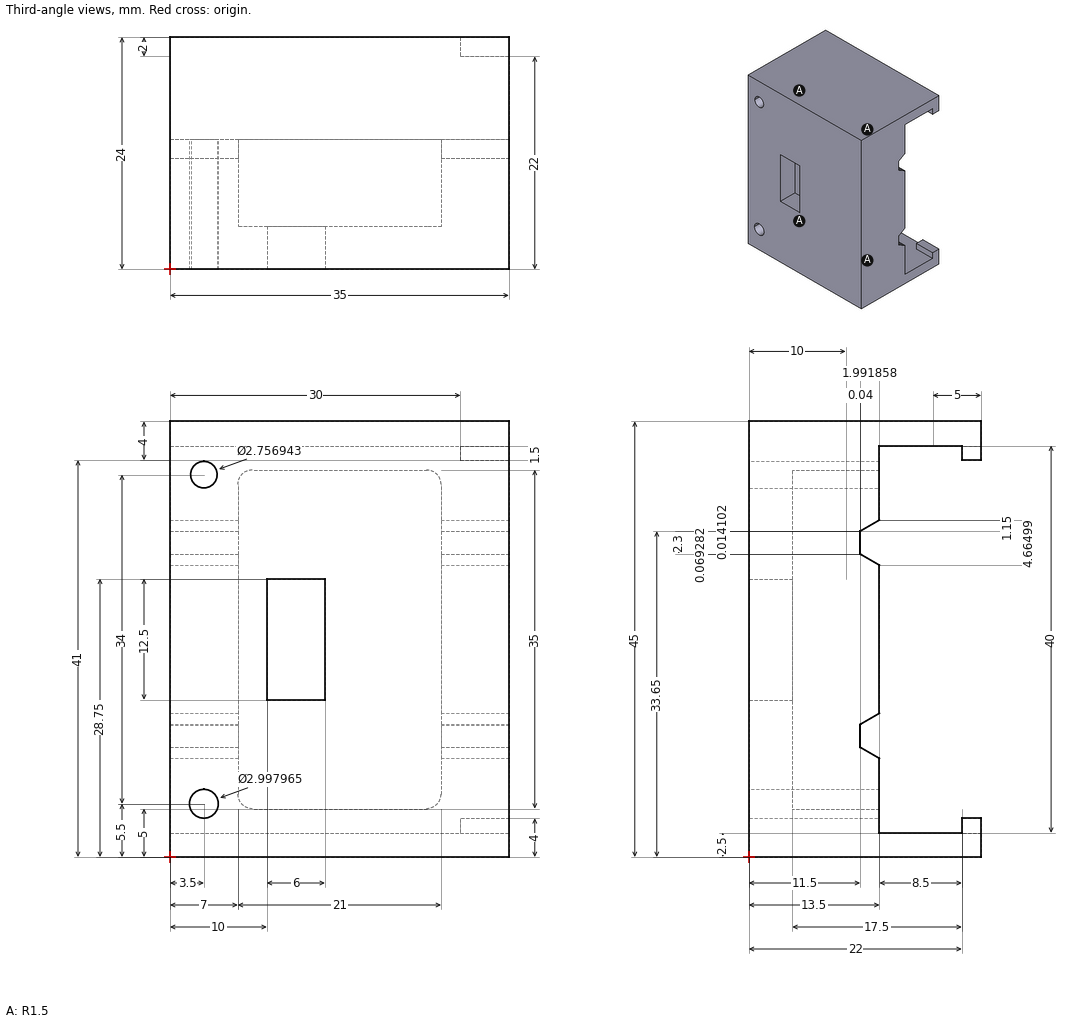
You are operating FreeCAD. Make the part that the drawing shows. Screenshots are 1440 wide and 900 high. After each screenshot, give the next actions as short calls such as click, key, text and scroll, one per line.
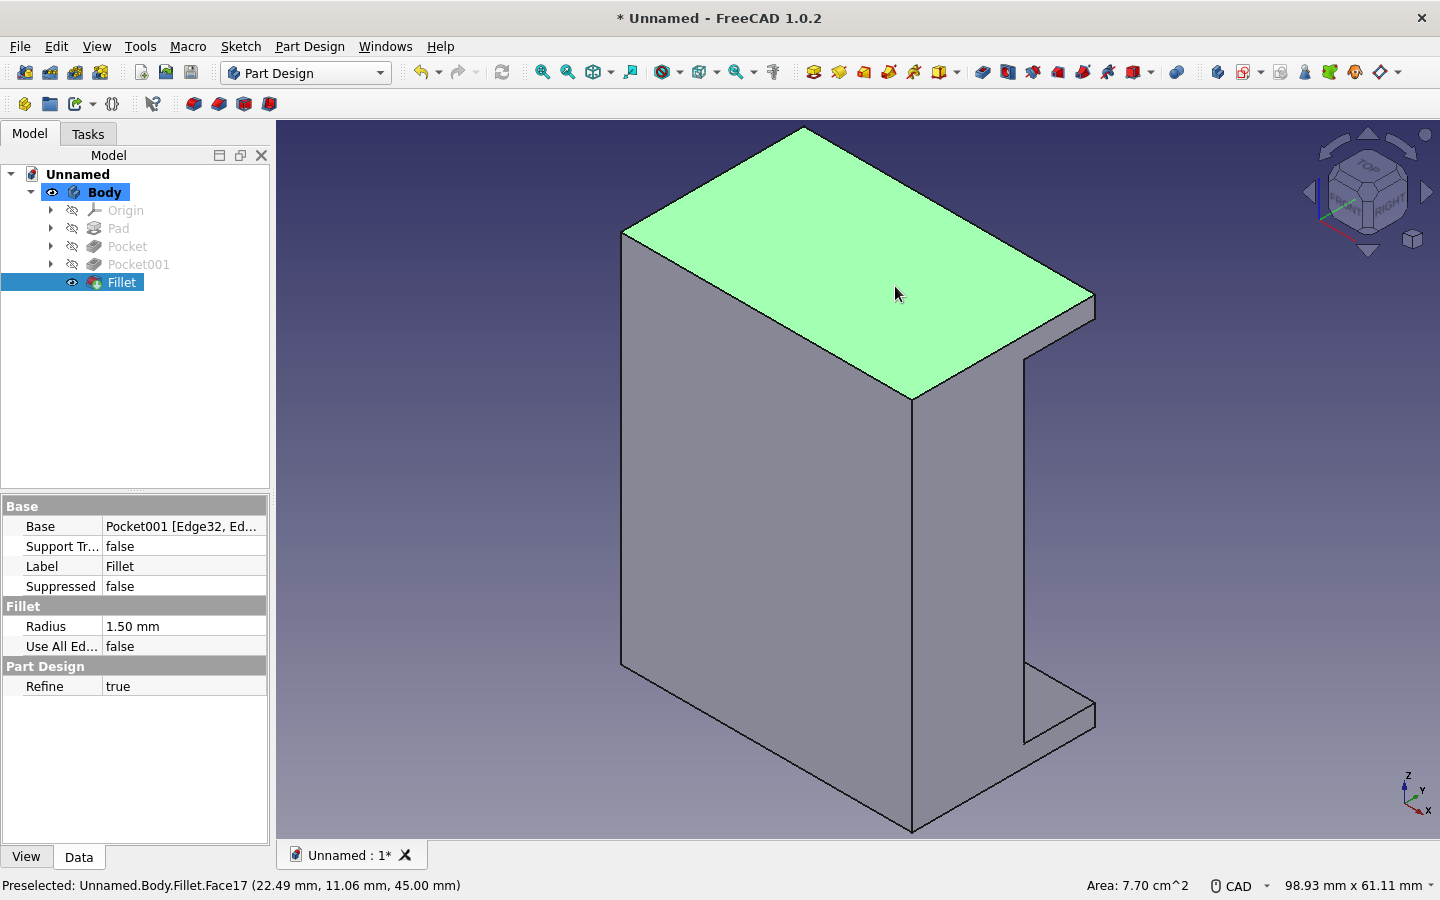
click(1242, 72)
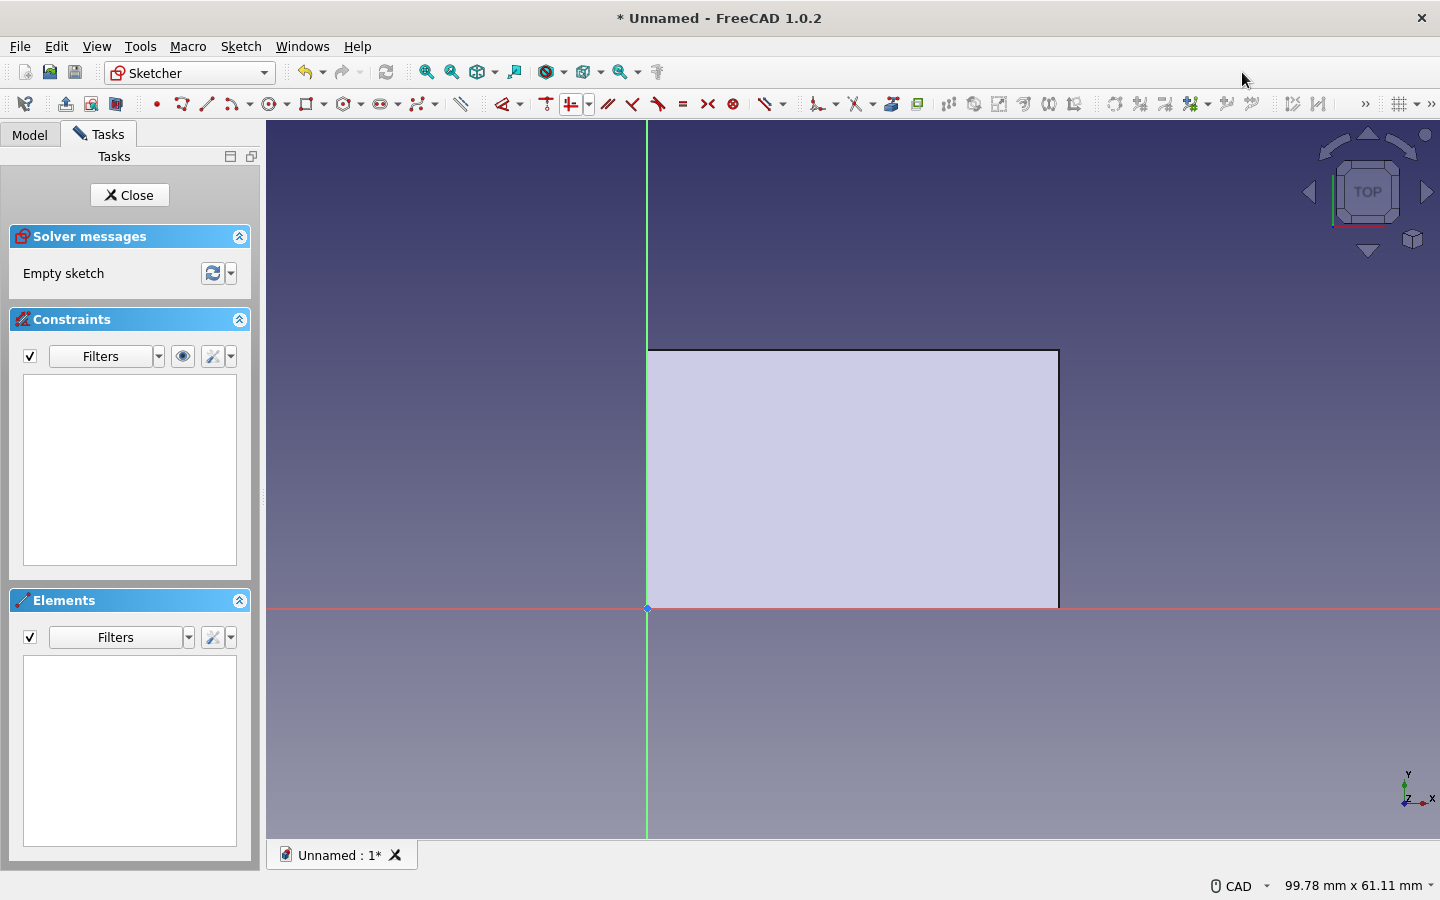
scroll(936, 453, up, 3)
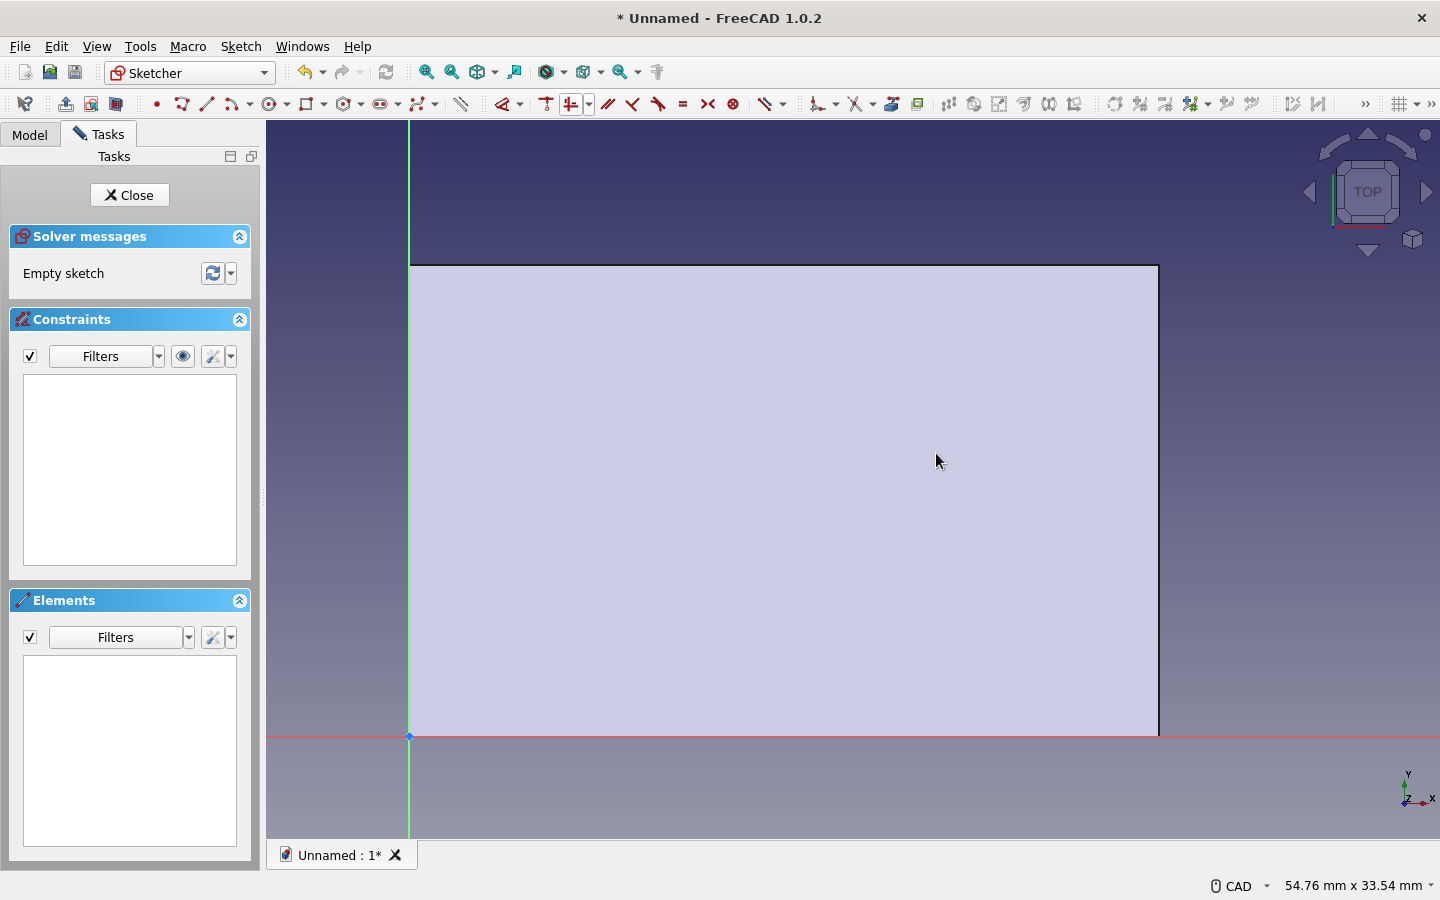
click(306, 104)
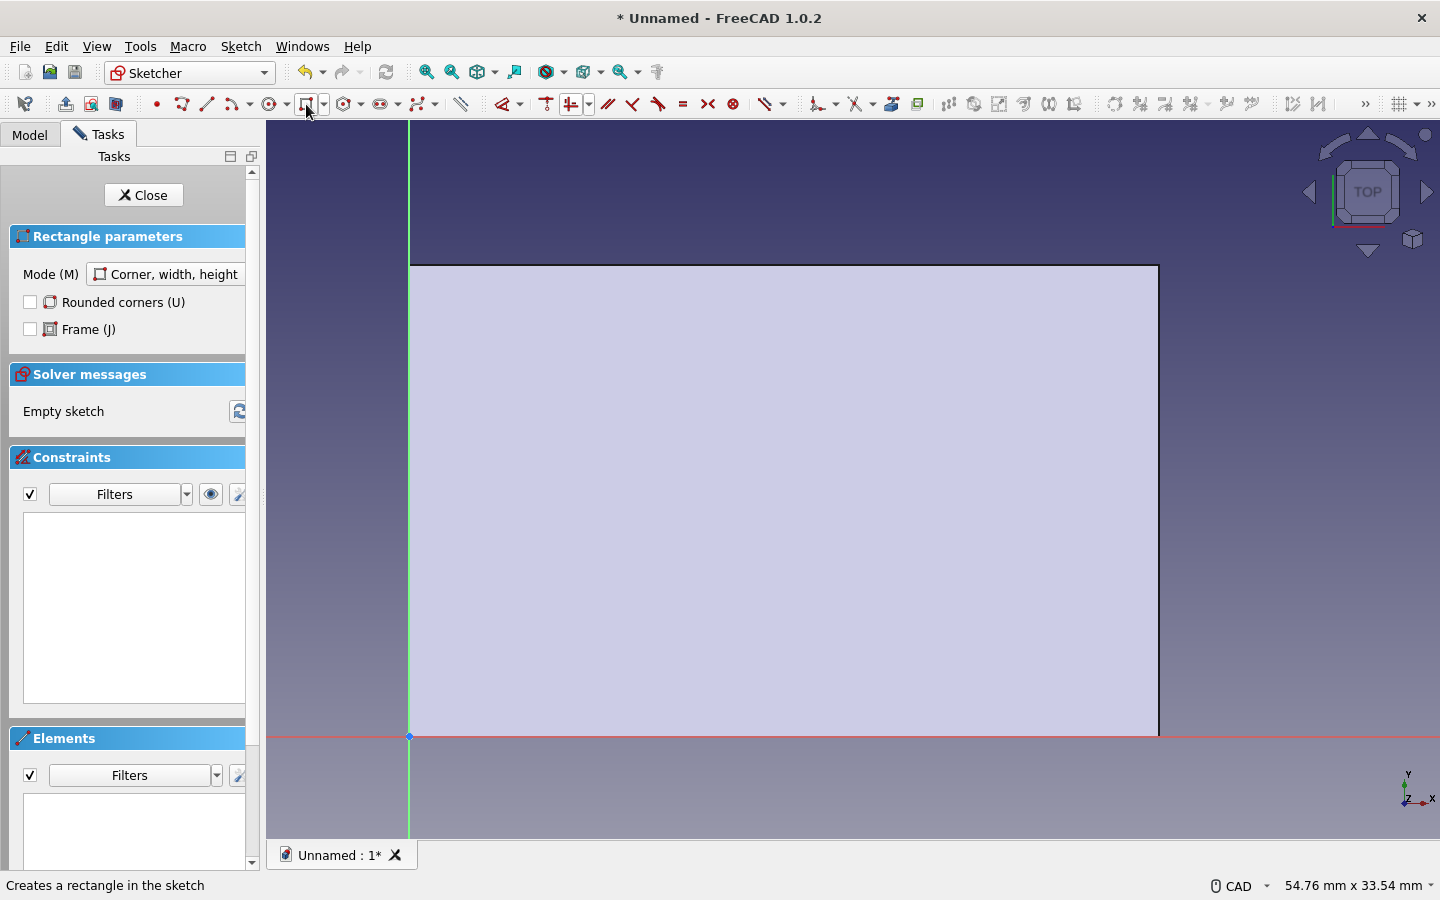
click(409, 222)
click(1159, 265)
key(Escape)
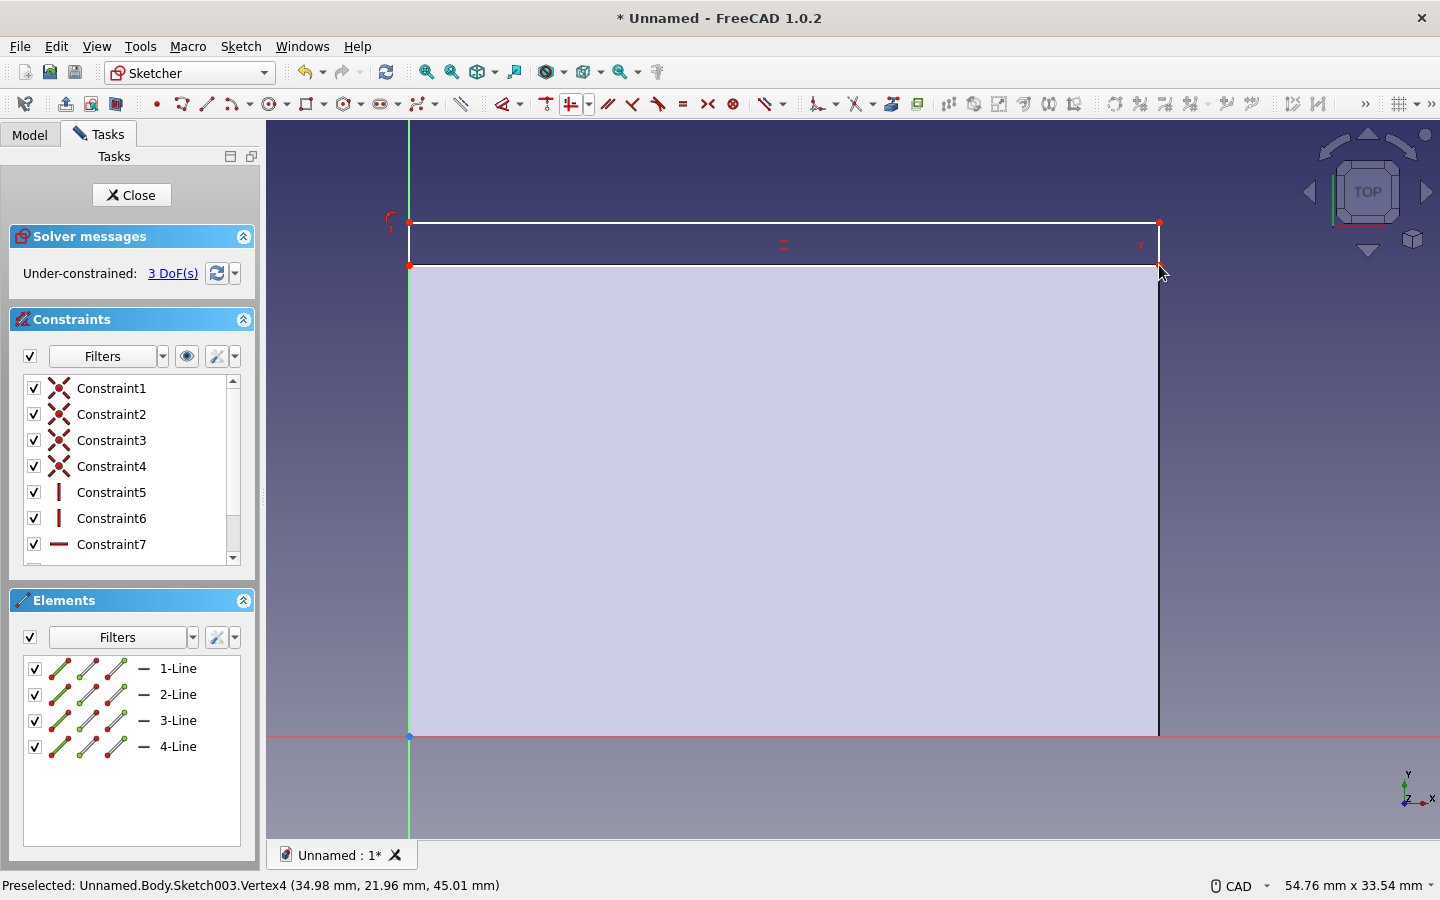
click(502, 104)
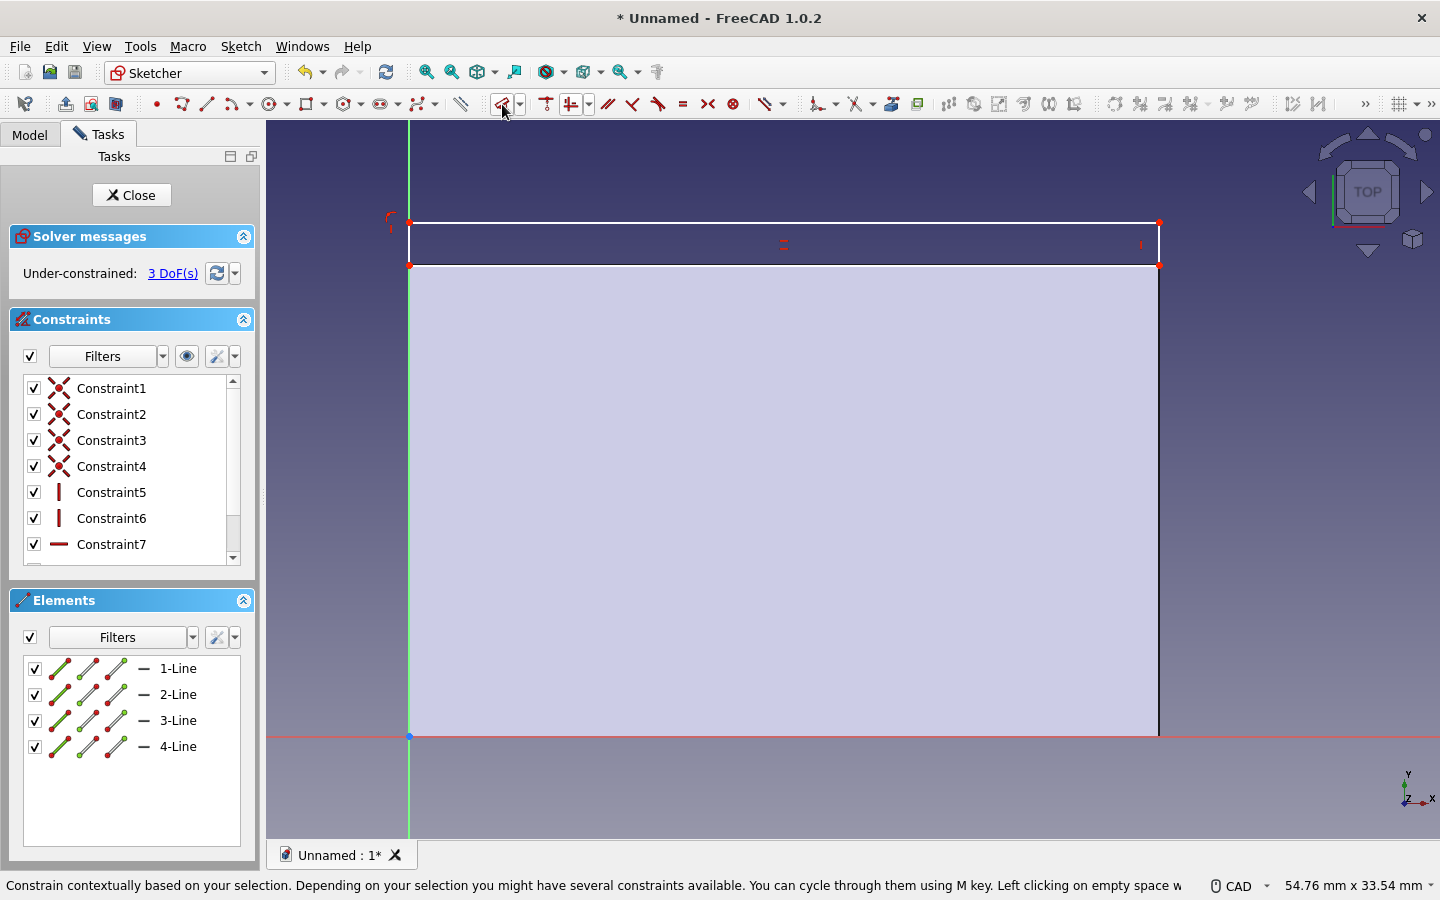
click(409, 236)
click(375, 244)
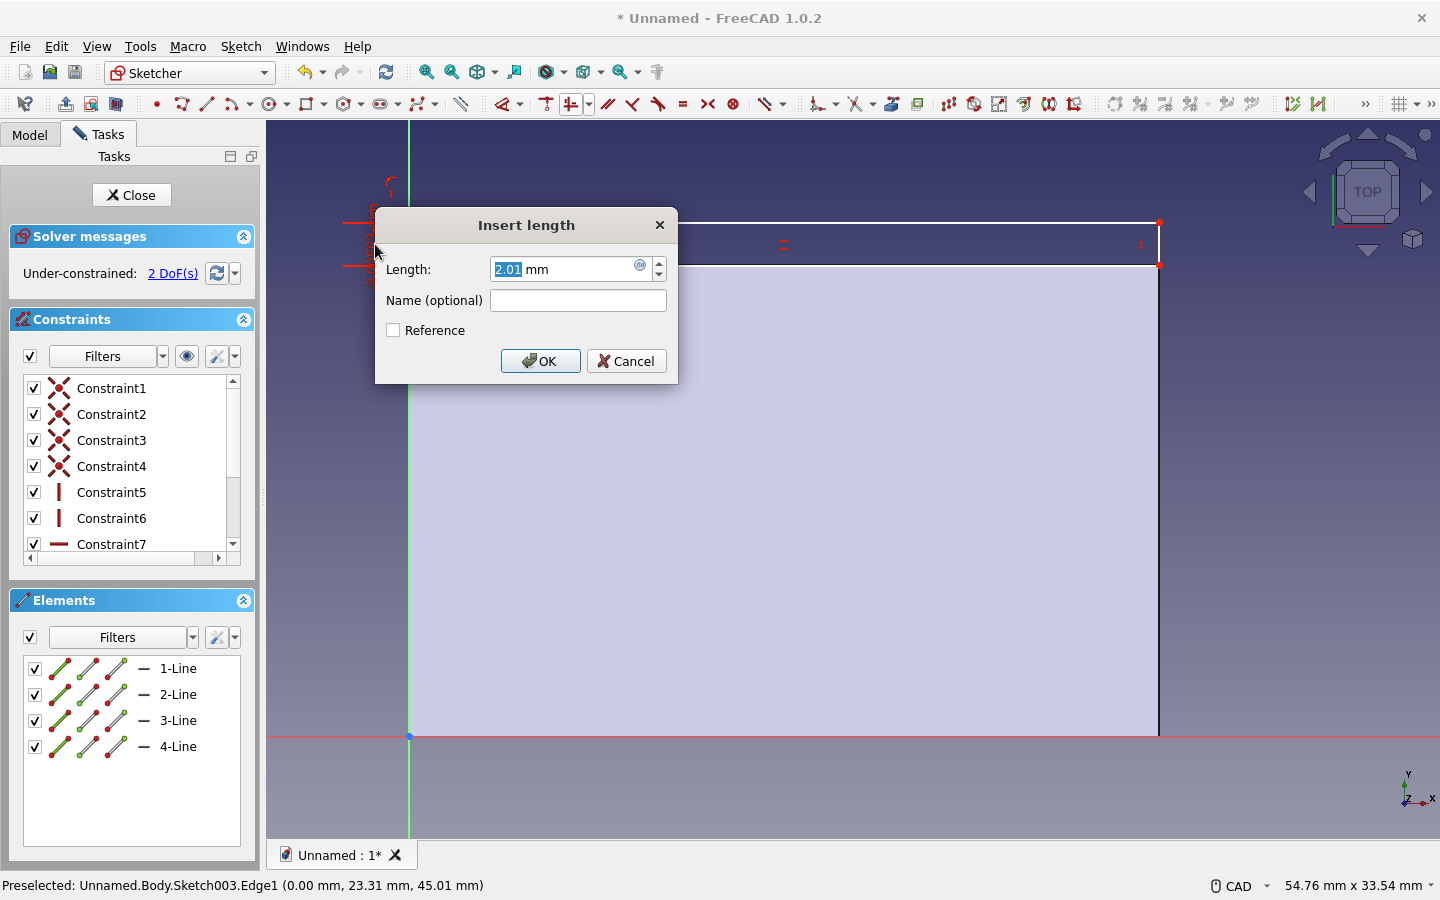
text(2)
key(Return)